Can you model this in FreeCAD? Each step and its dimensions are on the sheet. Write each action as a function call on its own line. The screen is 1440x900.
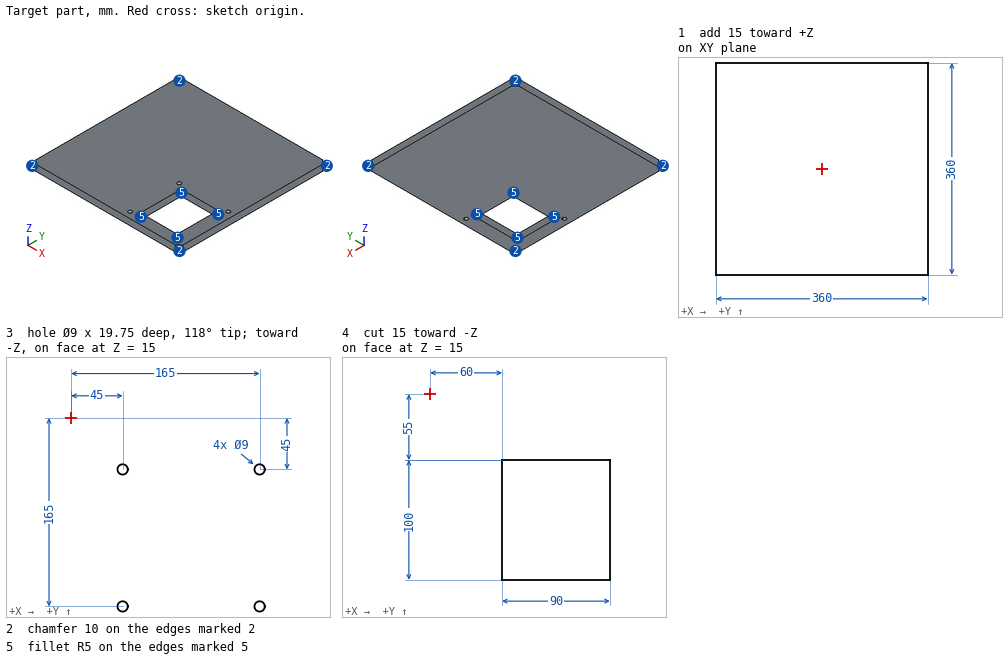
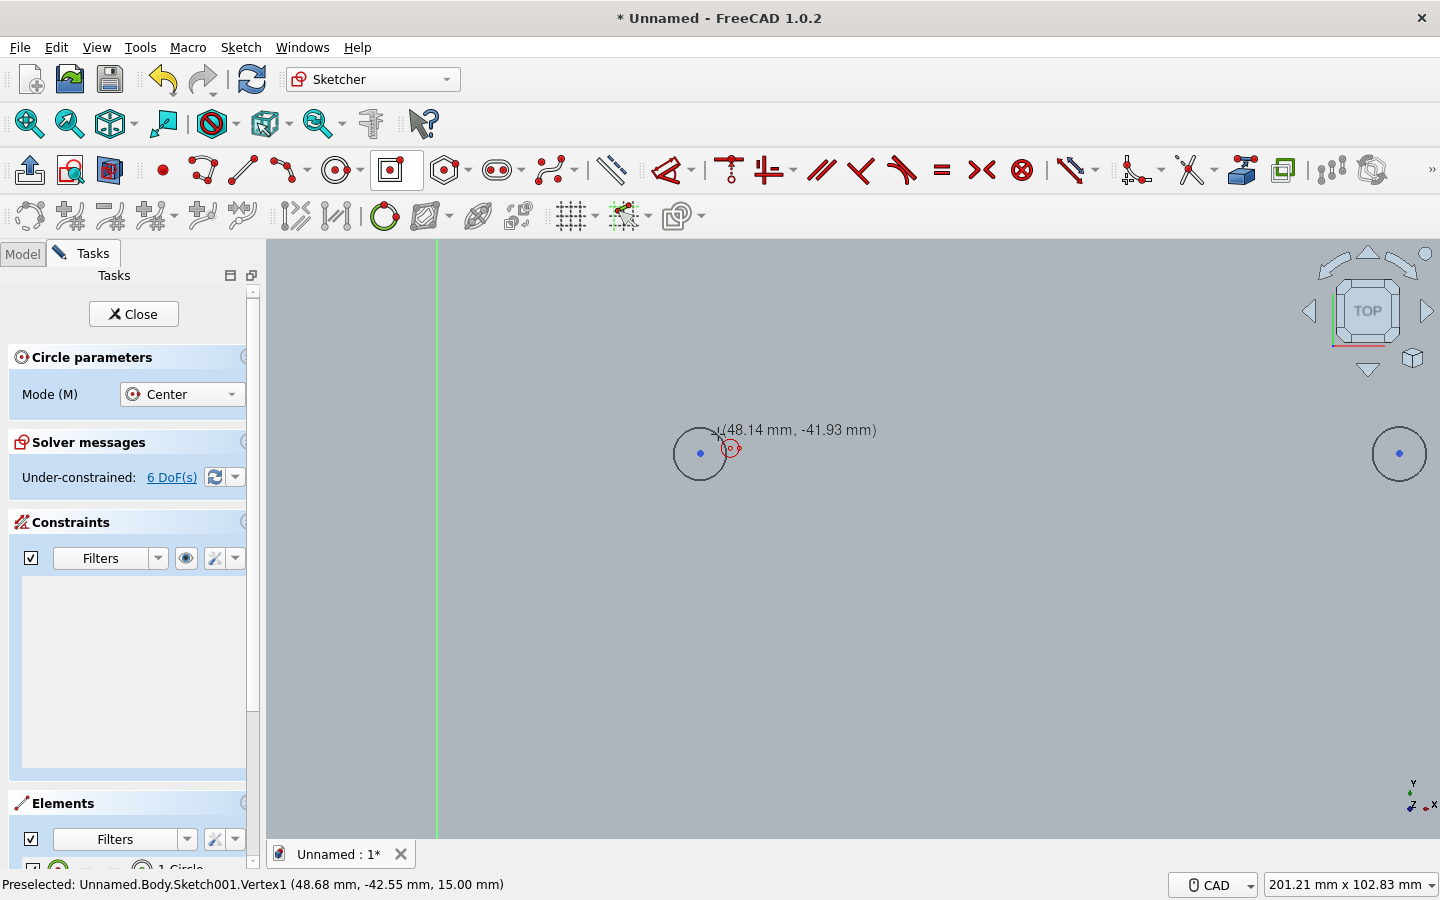
scroll(699, 454, down, 5)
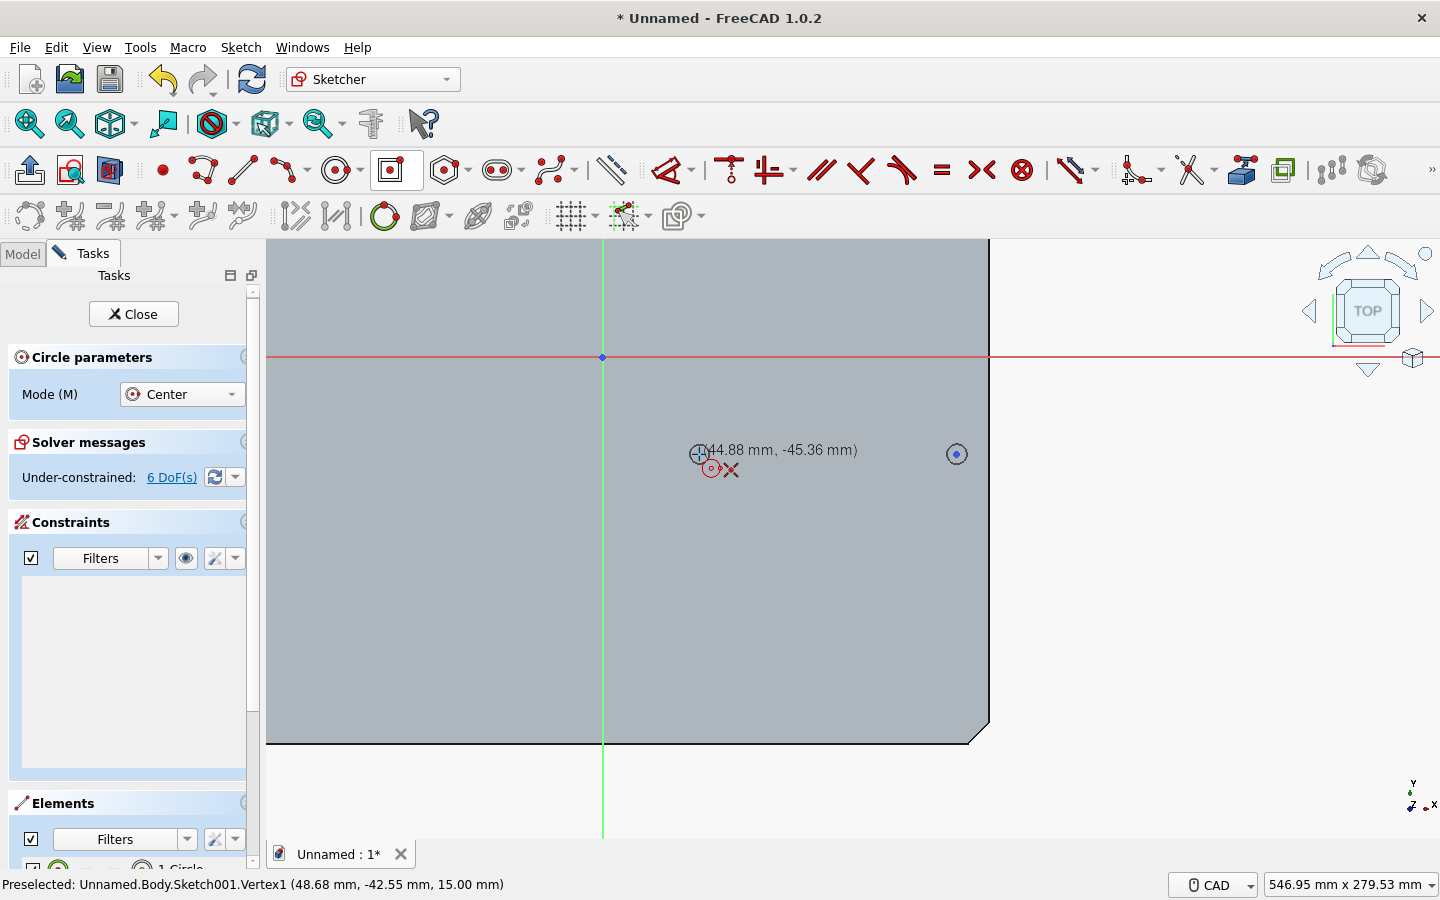
scroll(699, 711, up, 5)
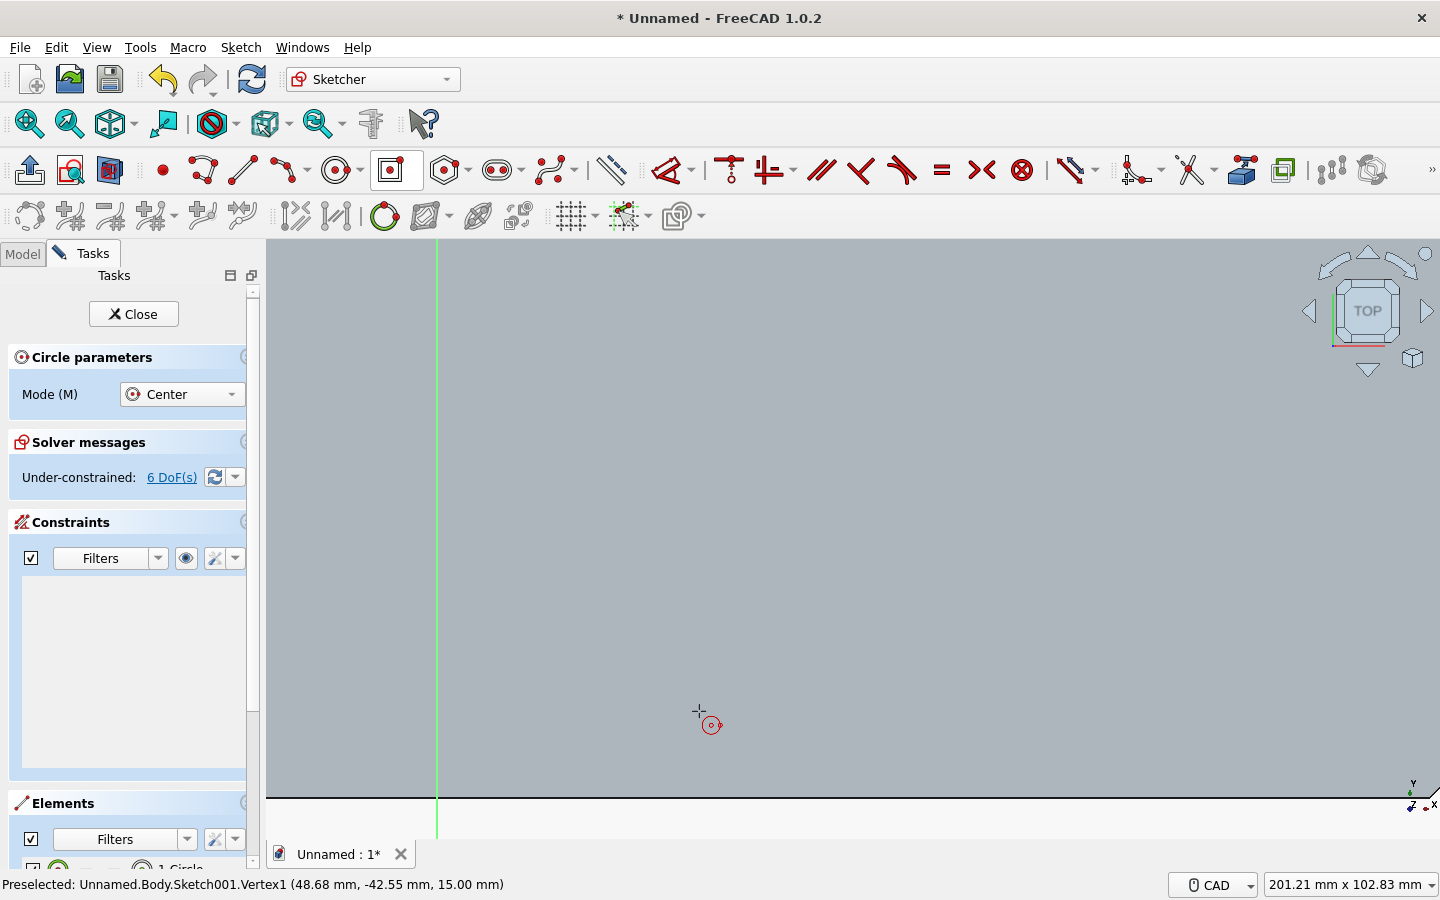
click(700, 711)
click(718, 692)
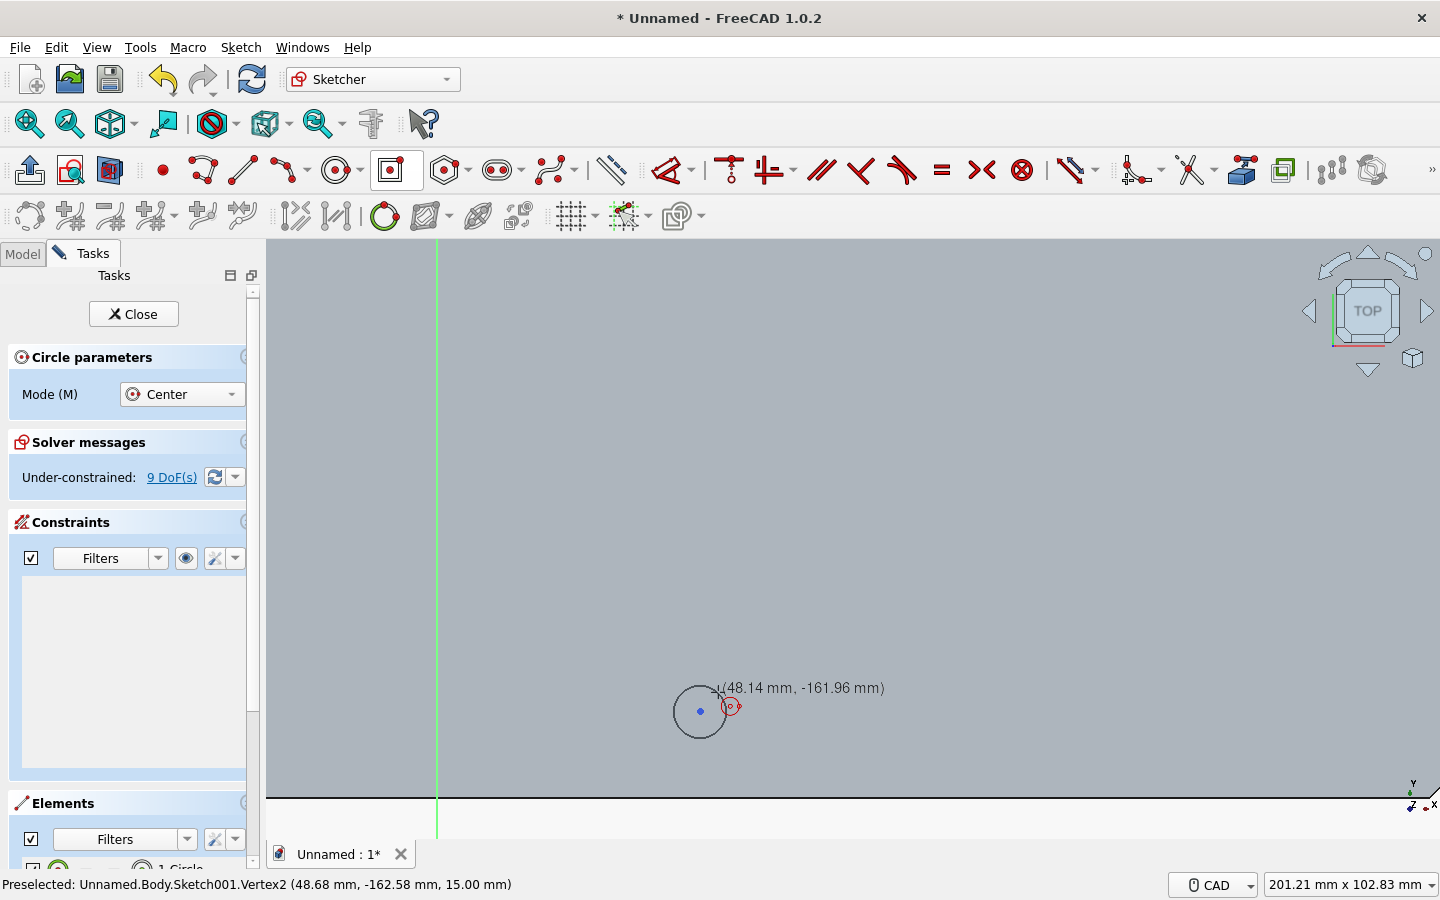
scroll(699, 712, down, 5)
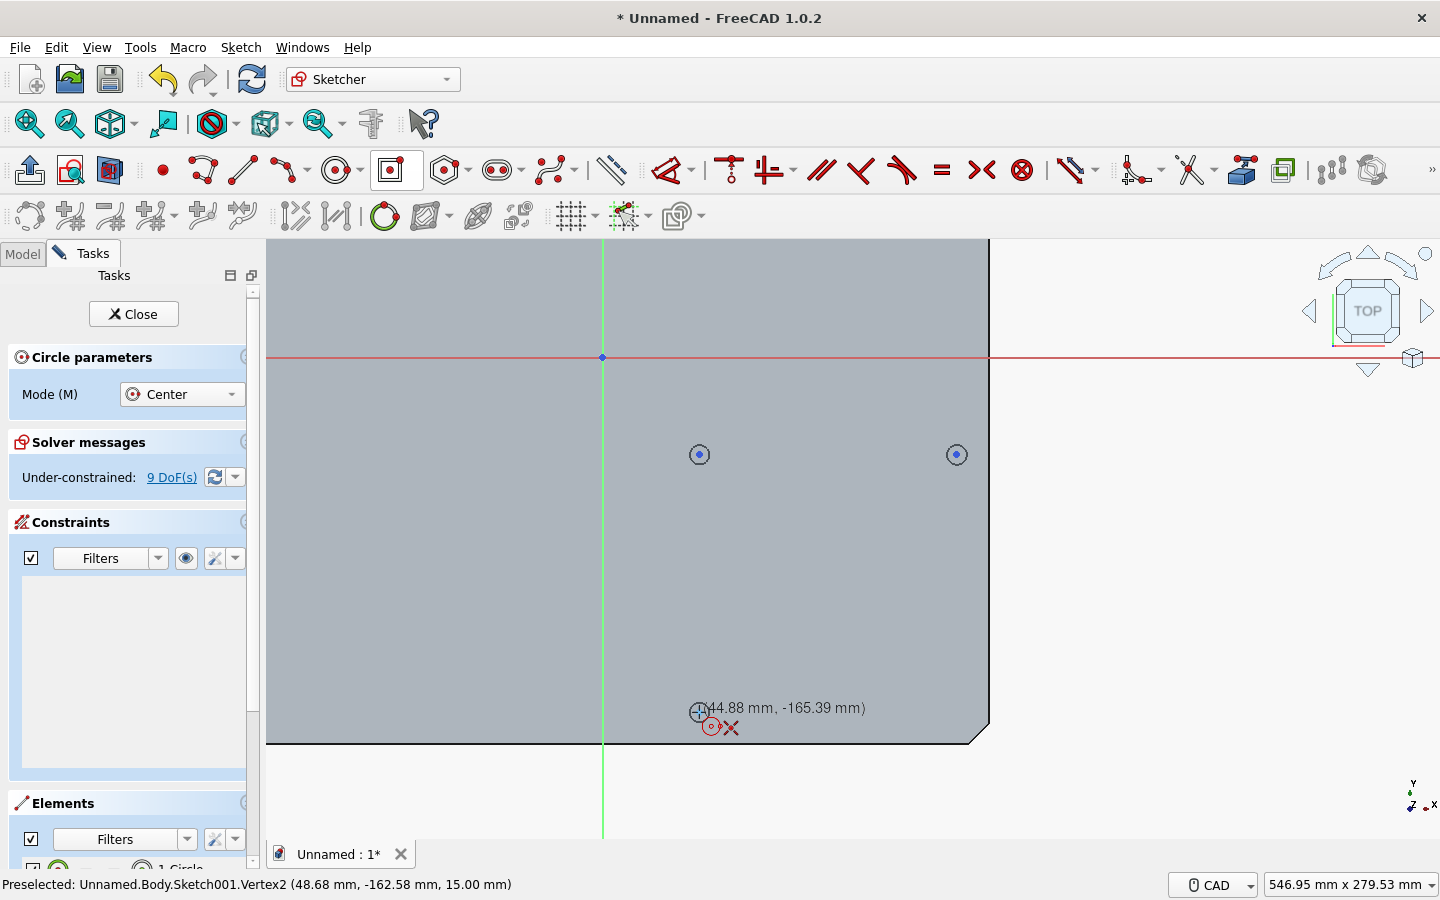
scroll(957, 712, up, 5)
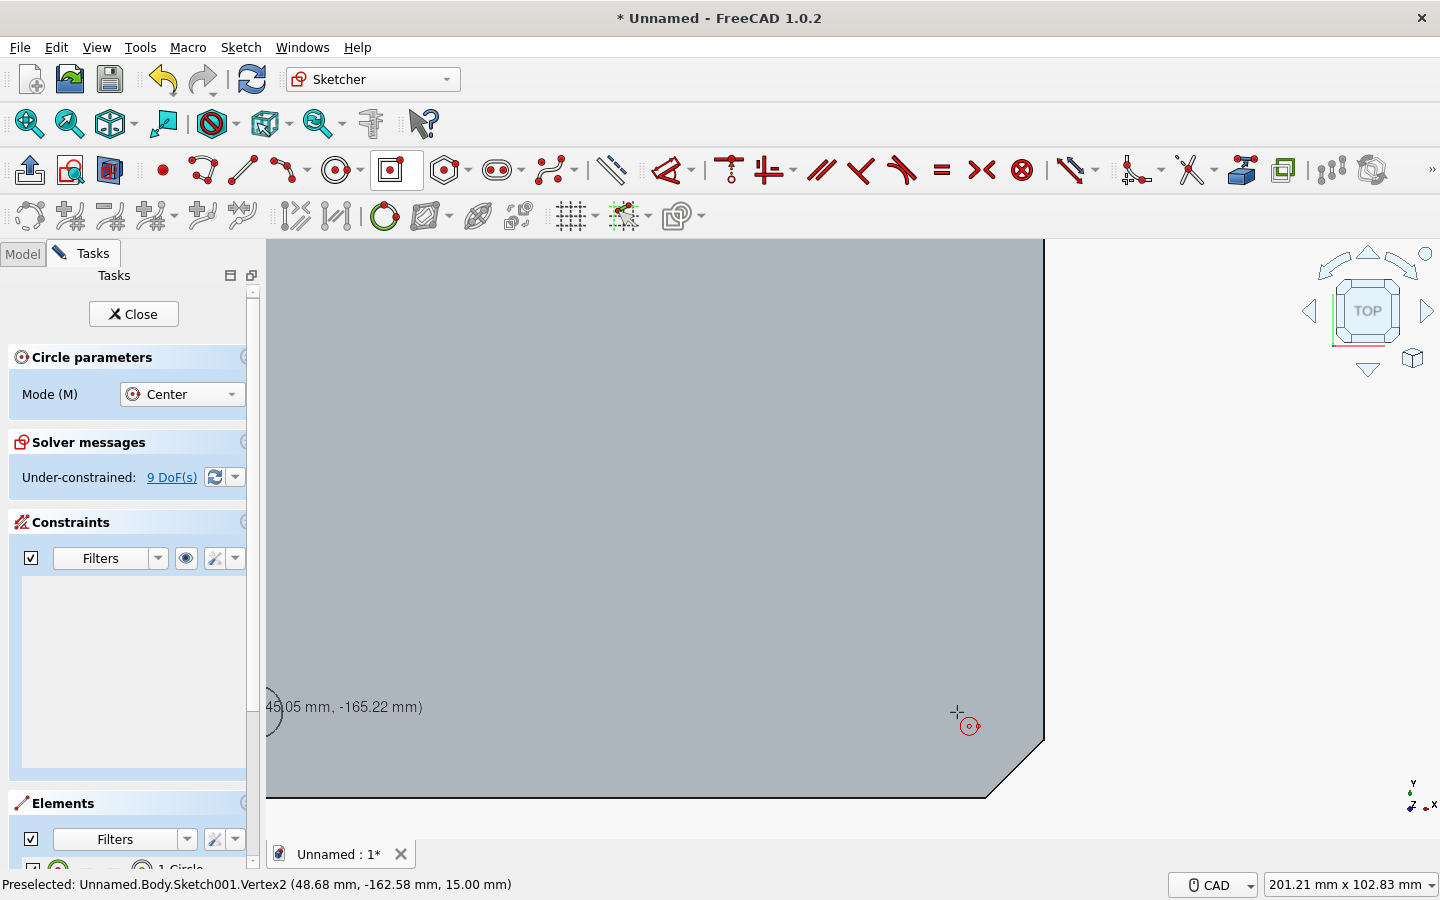
click(956, 711)
click(975, 692)
key(Escape)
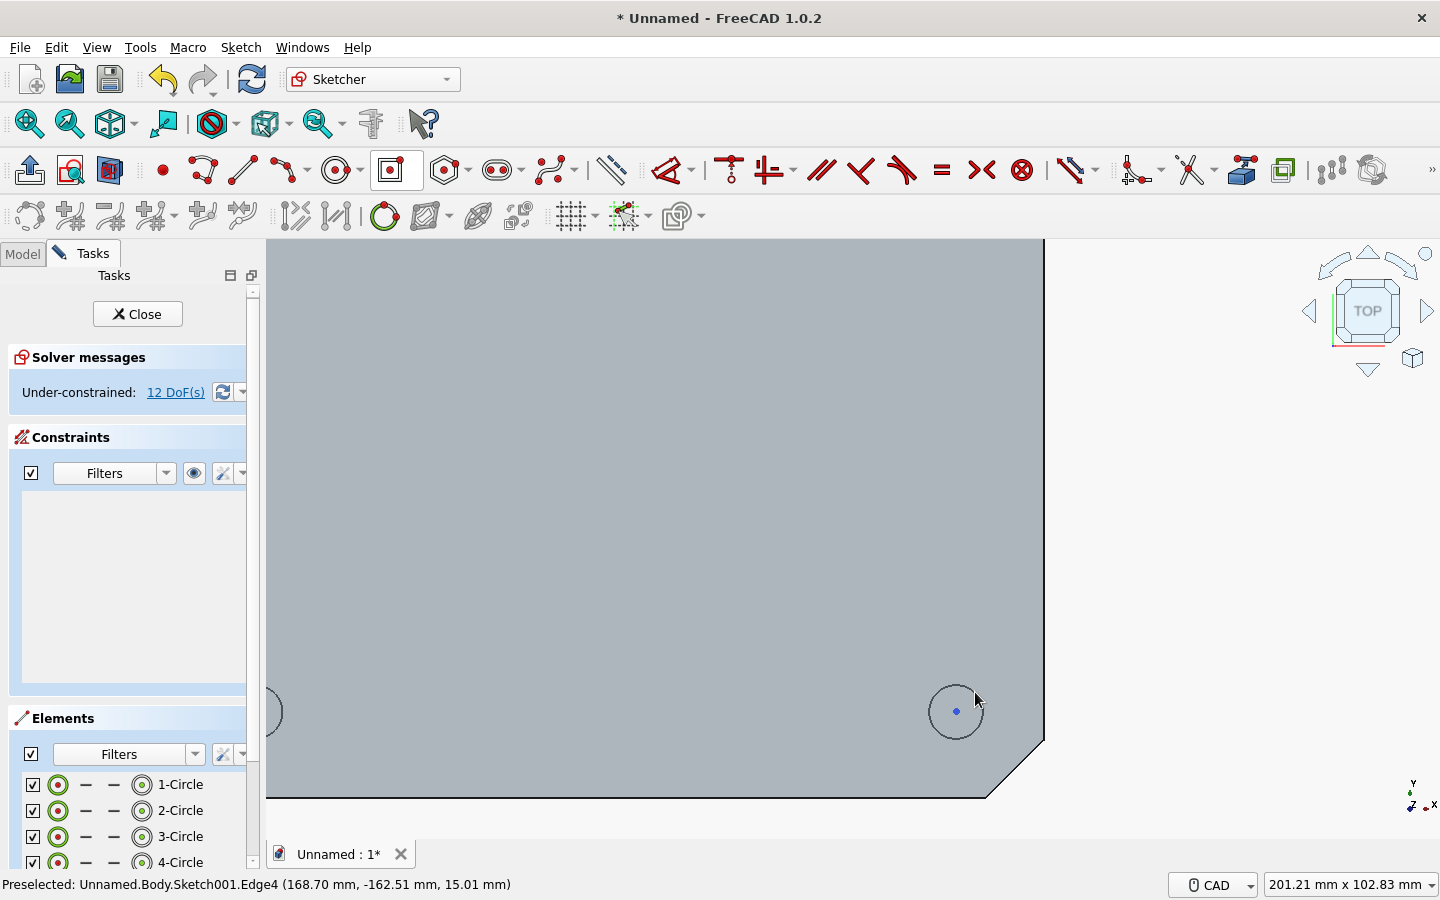
scroll(957, 712, down, 5)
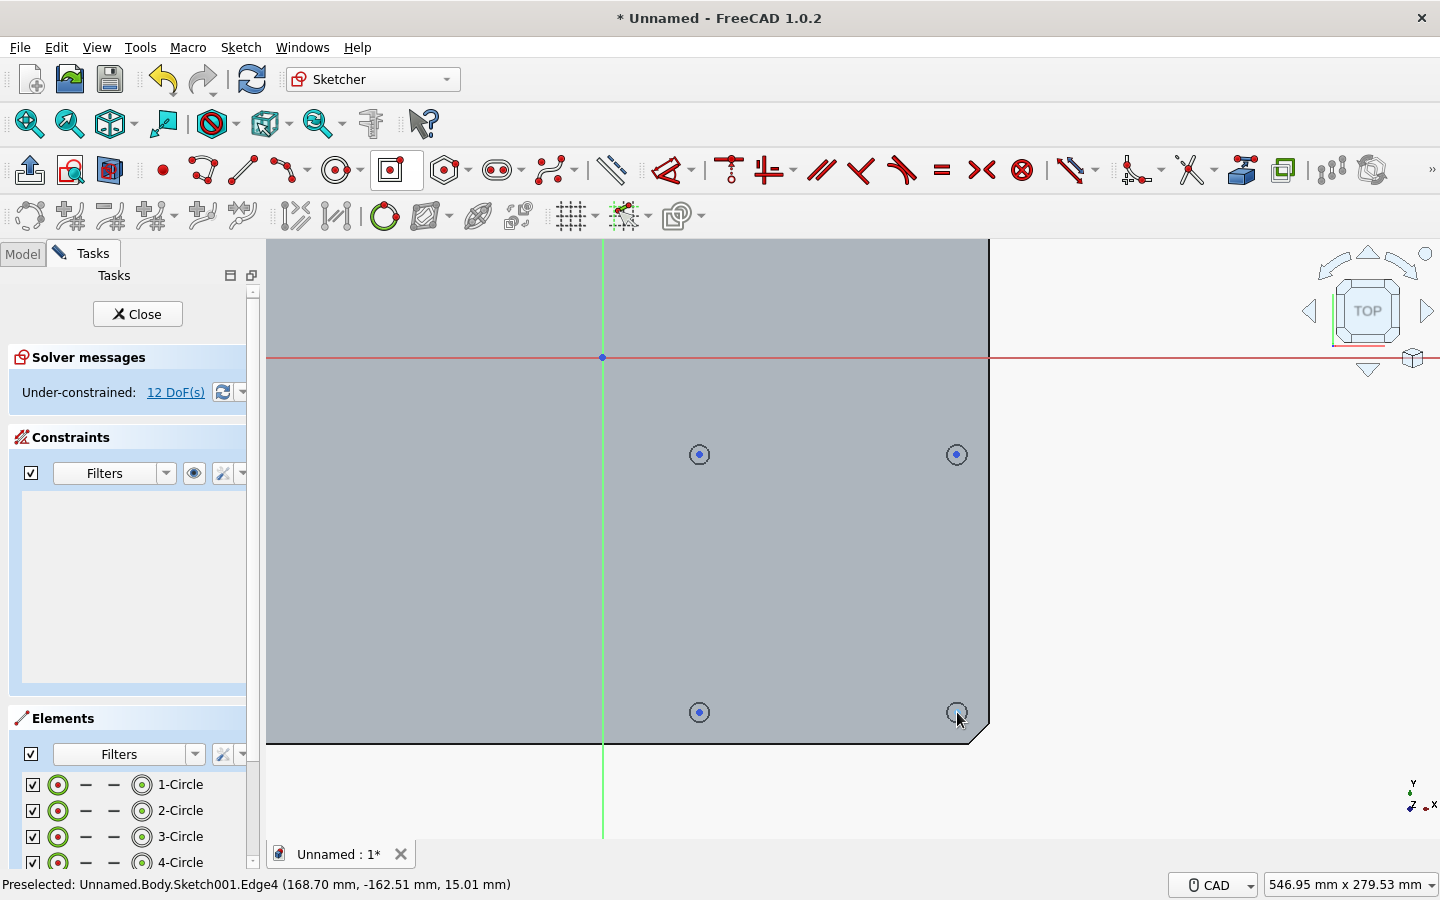
scroll(964, 448, up, 2)